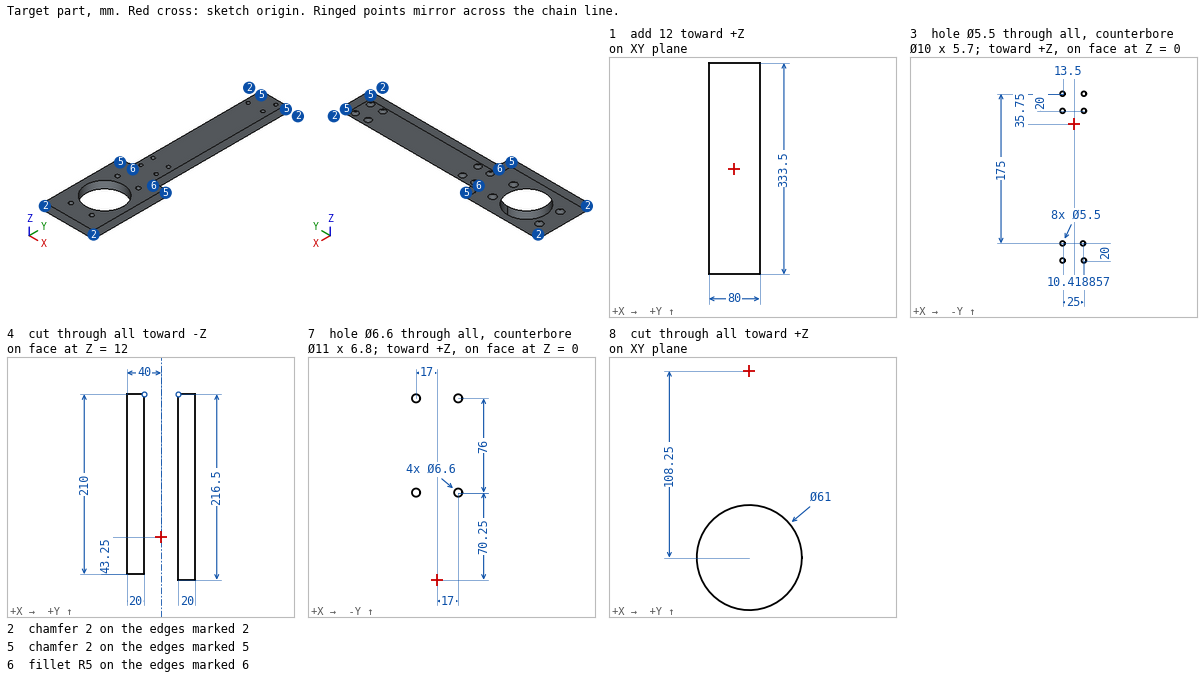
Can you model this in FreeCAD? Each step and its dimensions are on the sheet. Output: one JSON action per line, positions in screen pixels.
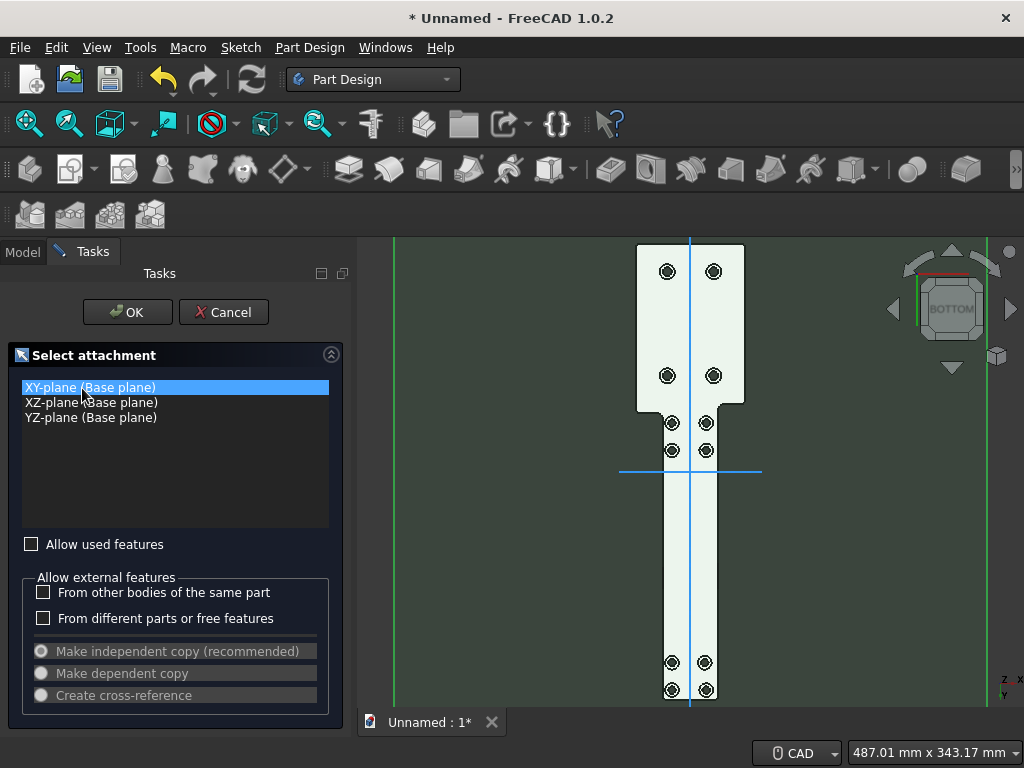
{"action": "left_click", "coordinate": [128, 312]}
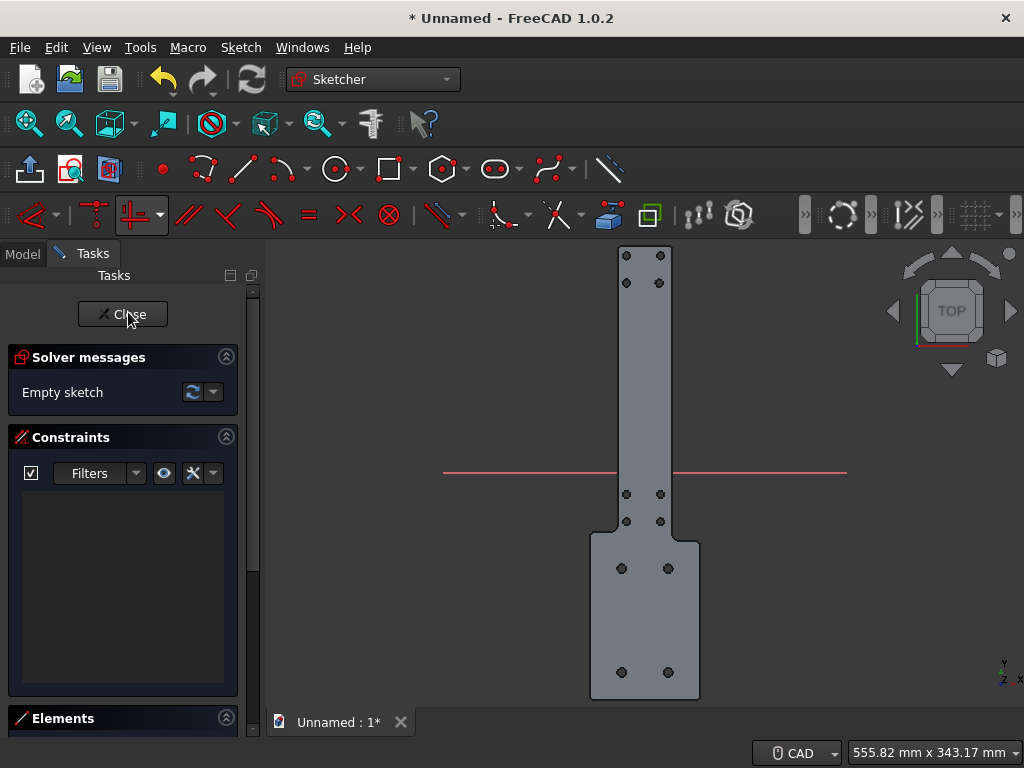
{"action": "key", "text": "q s"}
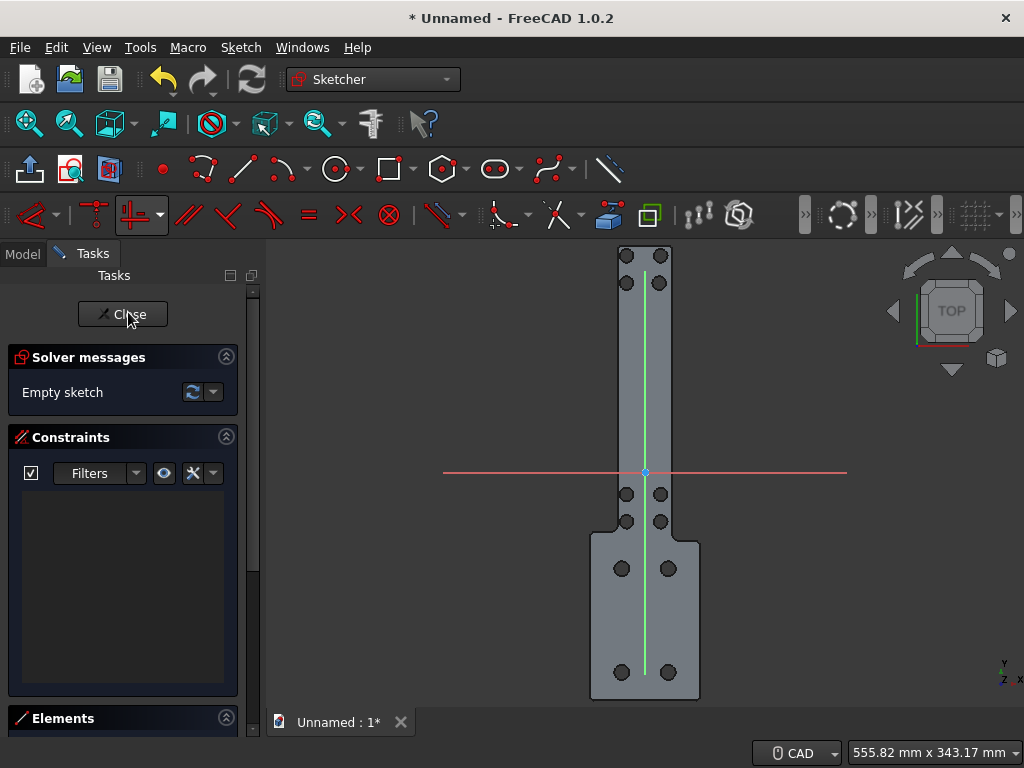
{"action": "scroll", "coordinate": [784, 679], "scroll_direction": "up", "scroll_amount": 2}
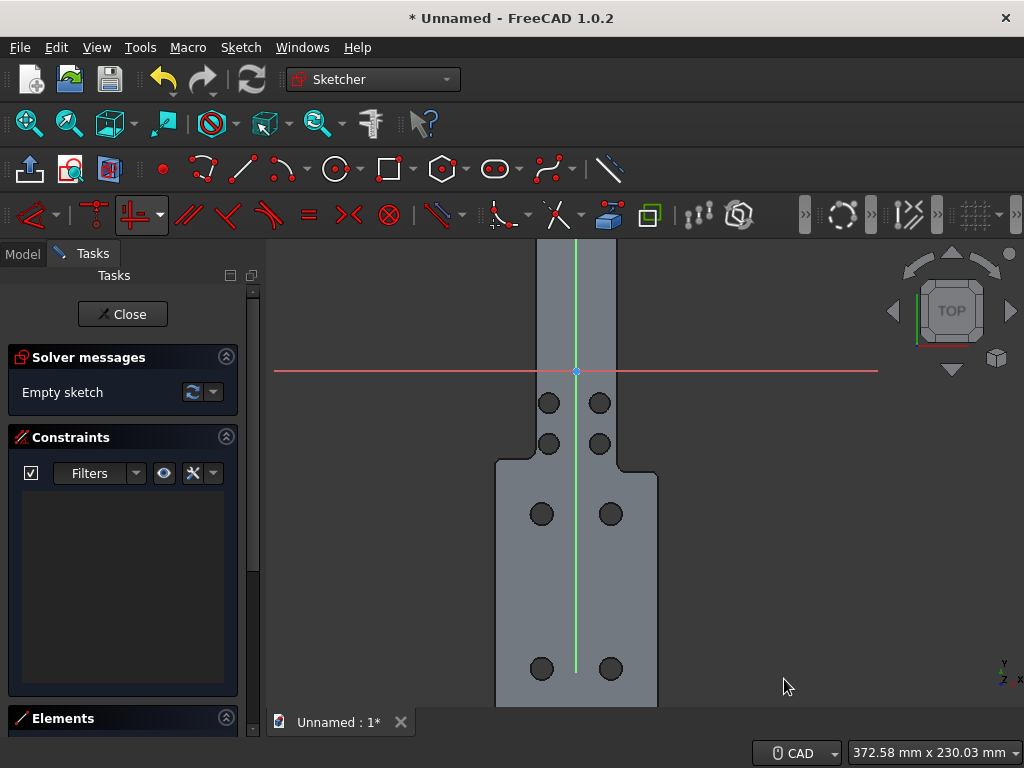
{"action": "left_click", "coordinate": [336, 170]}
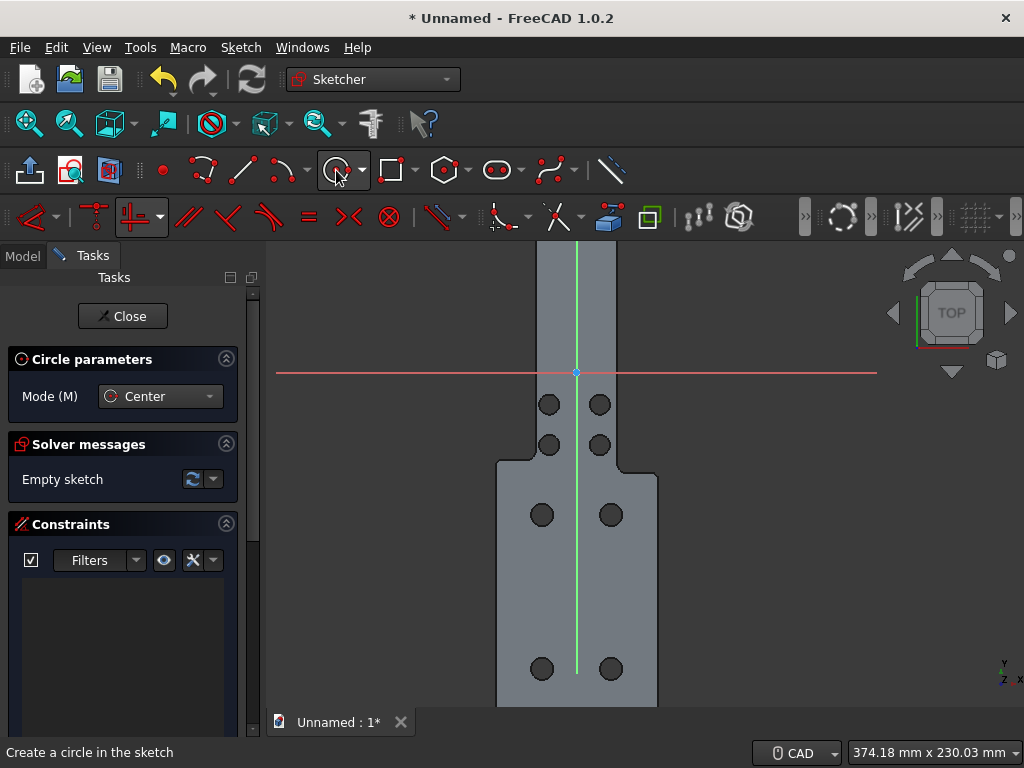
{"action": "left_click", "coordinate": [577, 592]}
{"action": "left_click", "coordinate": [620, 548]}
{"action": "key", "text": "Escape"}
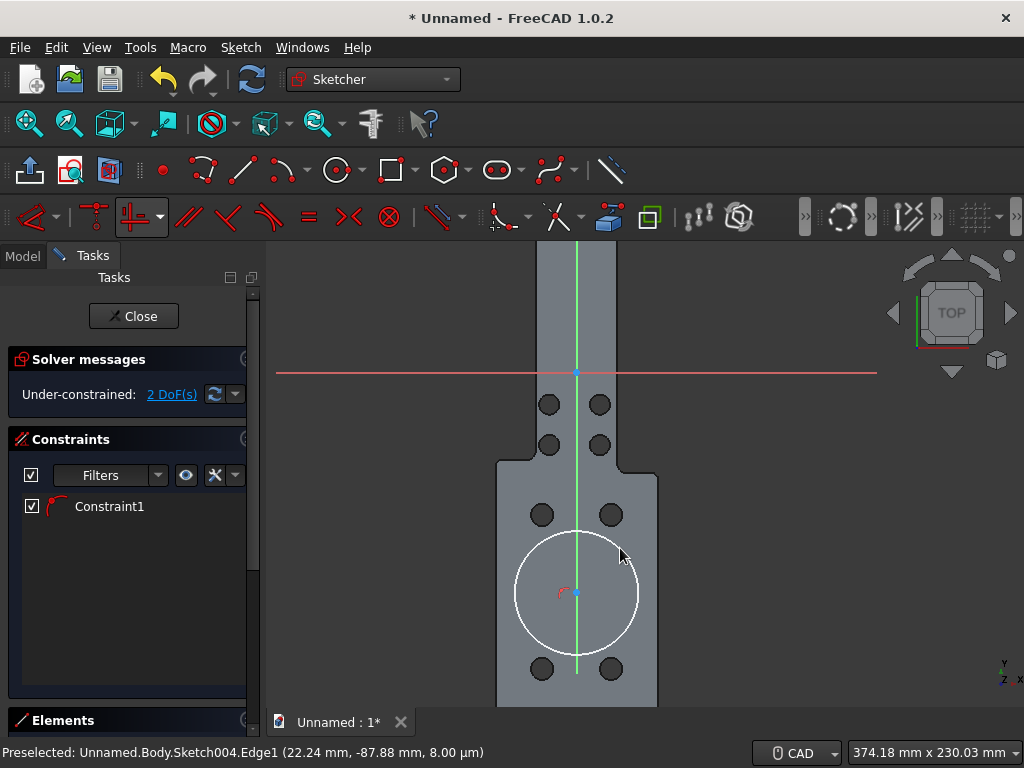
{"action": "key", "text": "d"}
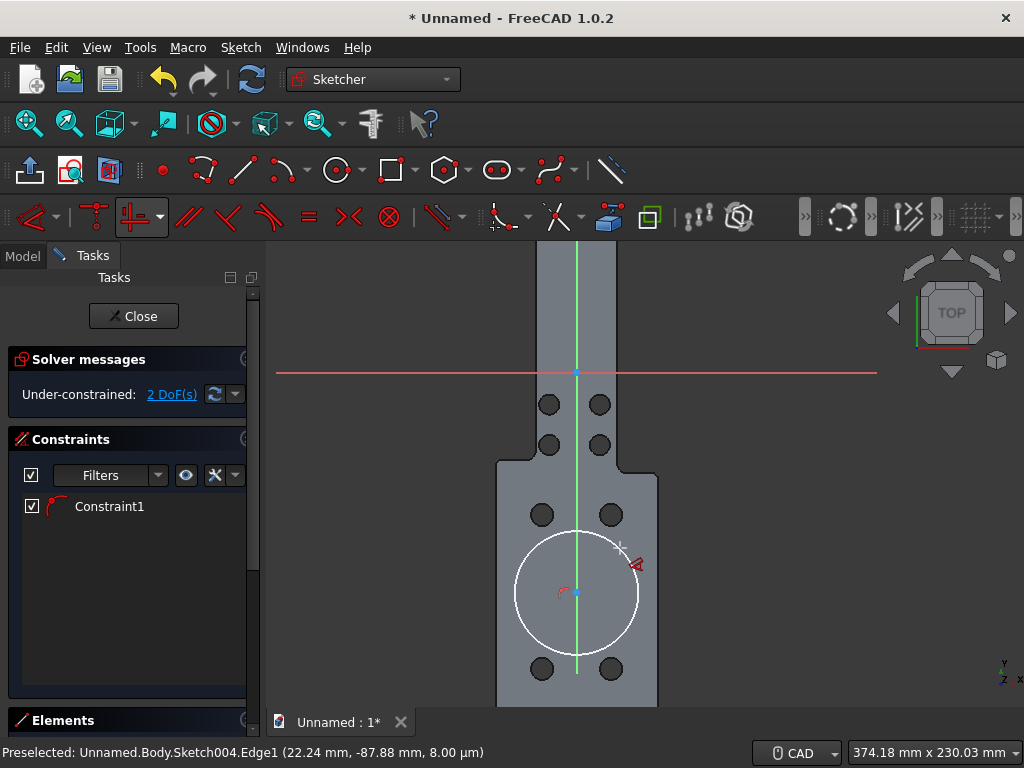
{"action": "left_click", "coordinate": [620, 549]}
{"action": "left_click", "coordinate": [642, 526]}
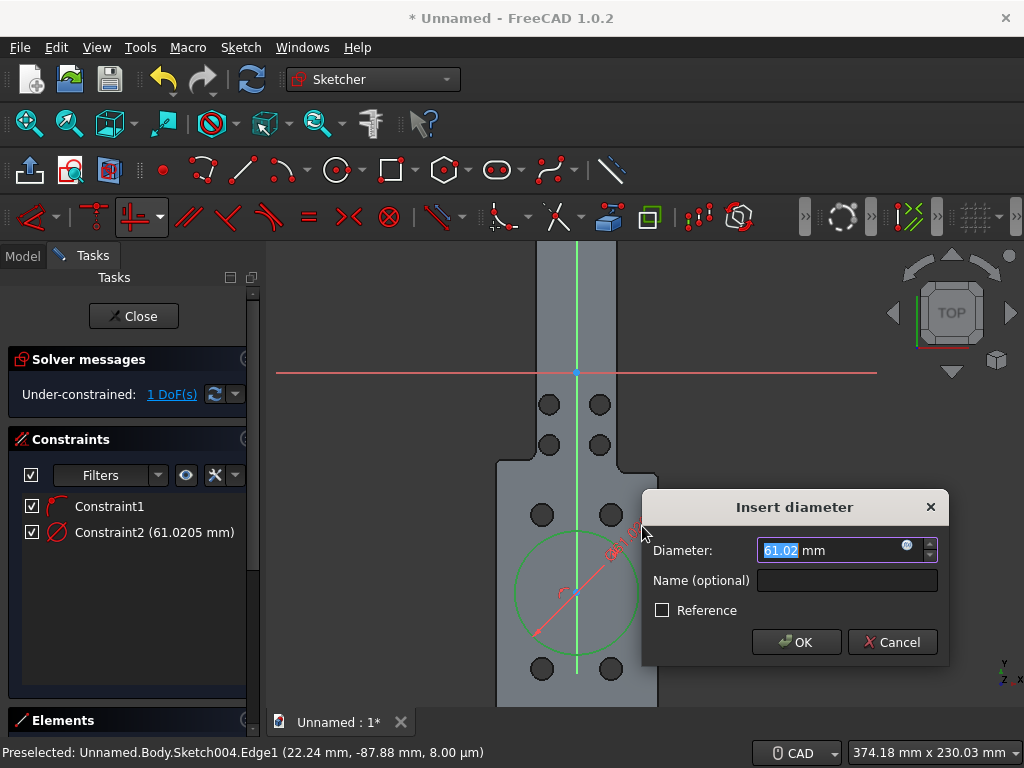
{"action": "type", "text": "61"}
{"action": "key", "text": "Return"}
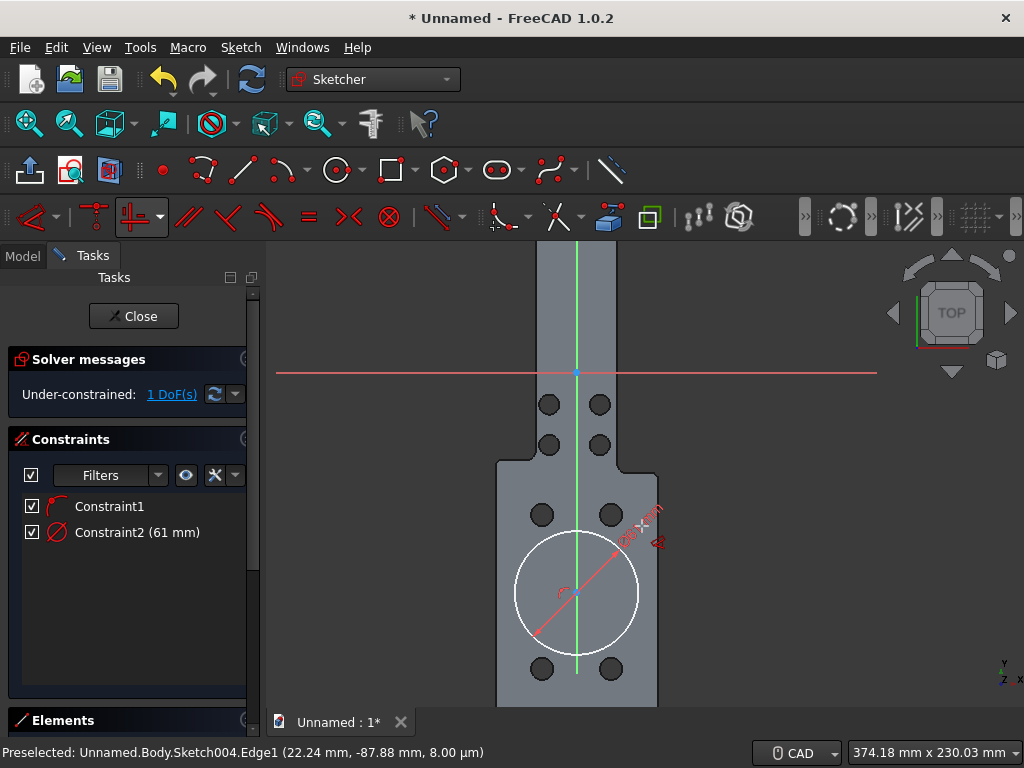
{"action": "left_click", "coordinate": [577, 593]}
{"action": "left_click", "coordinate": [611, 483]}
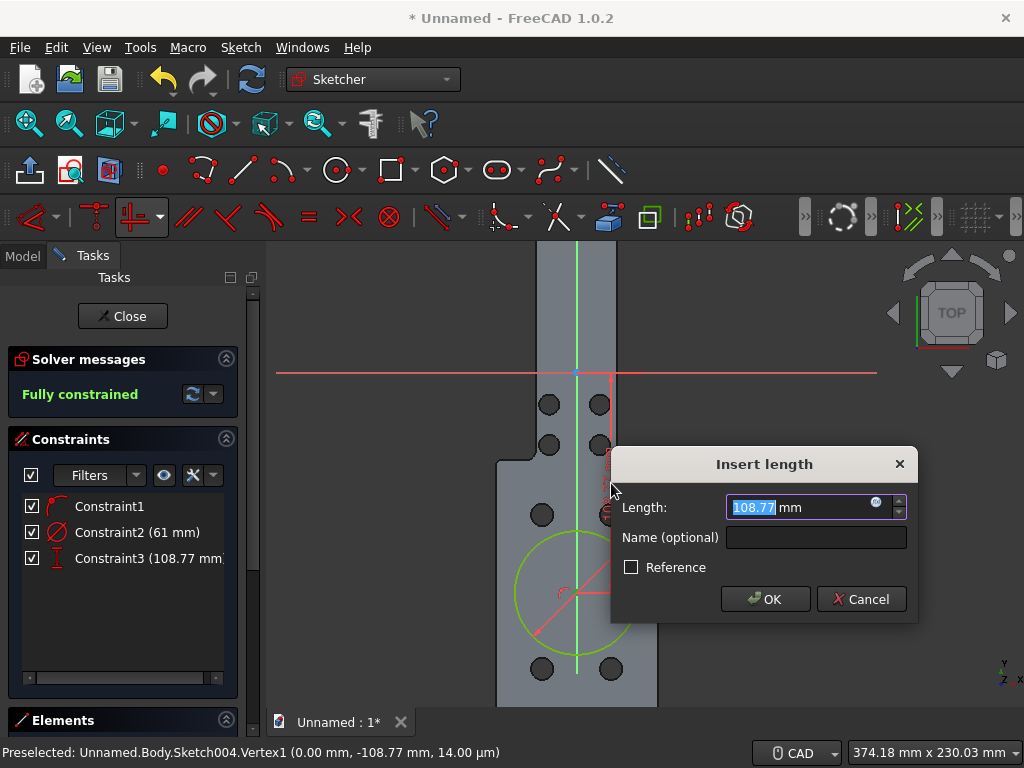
{"action": "type", "text": "108.25"}
{"action": "key", "text": "Return"}
{"action": "key", "text": "Escape"}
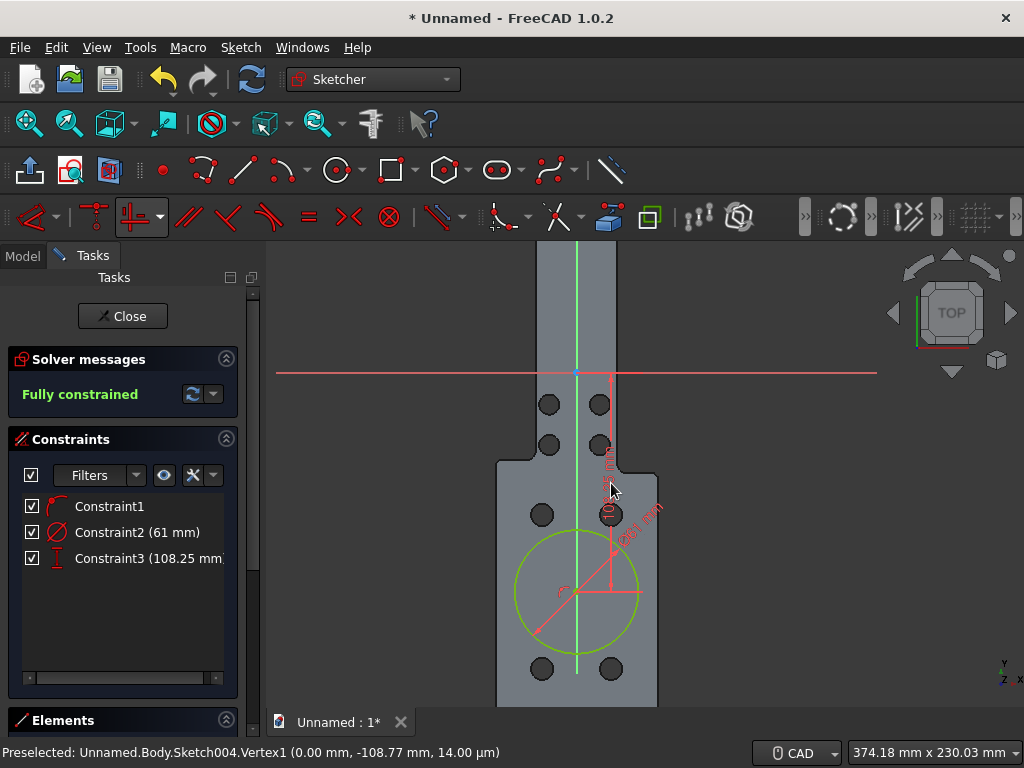
{"action": "left_click", "coordinate": [123, 316]}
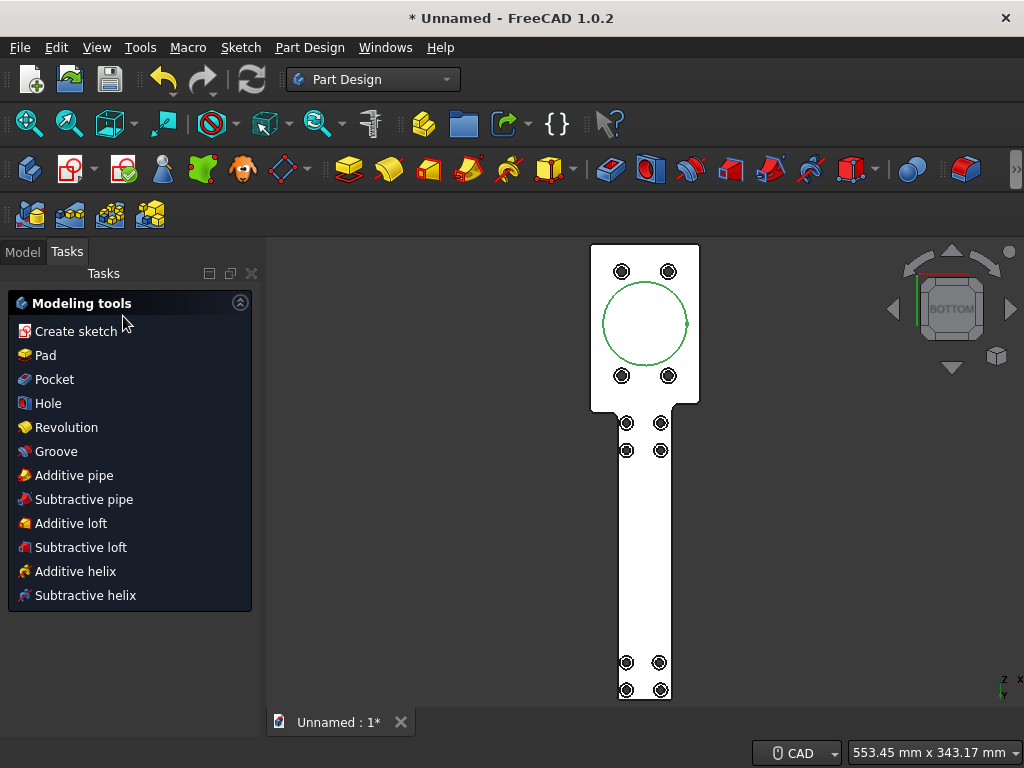
{"action": "left_click", "coordinate": [612, 170]}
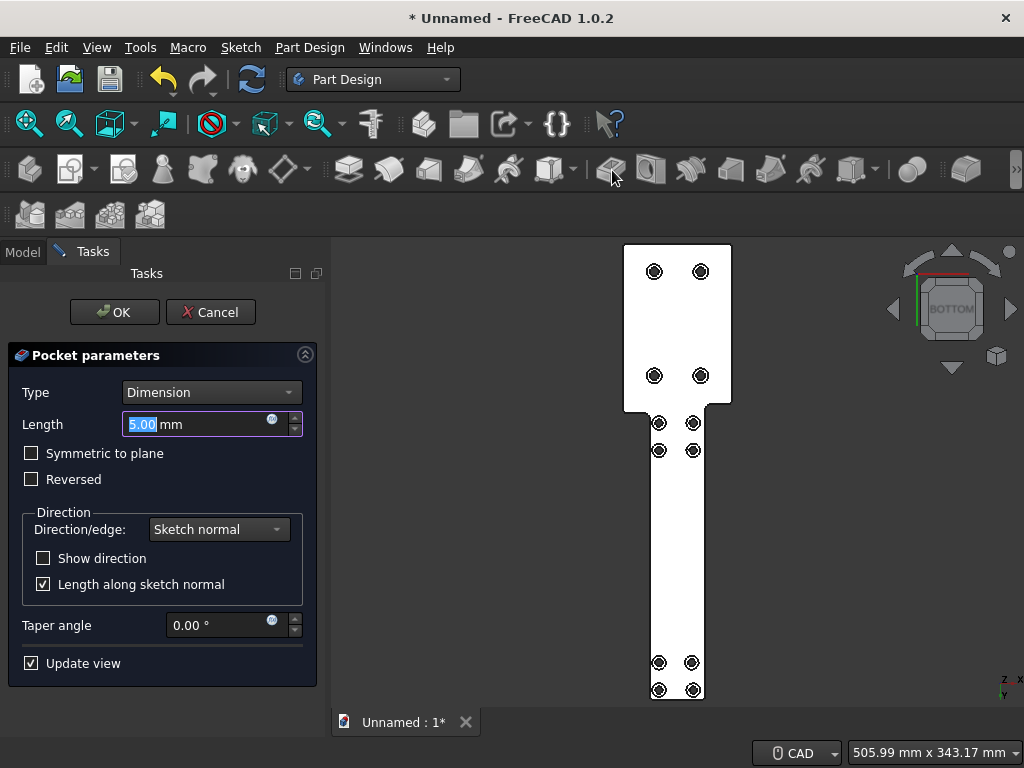
{"action": "left_click", "coordinate": [212, 392]}